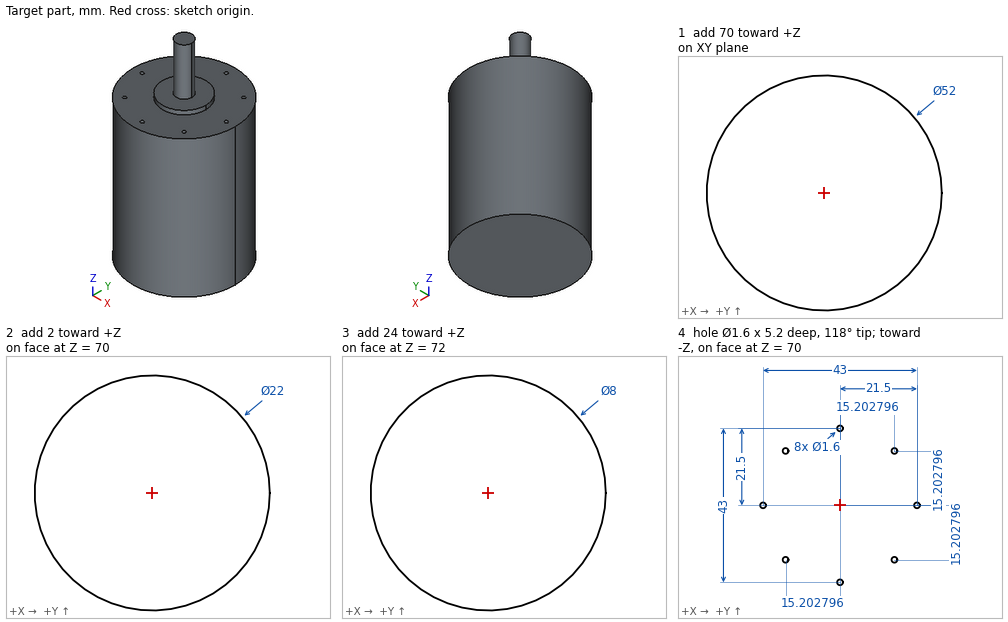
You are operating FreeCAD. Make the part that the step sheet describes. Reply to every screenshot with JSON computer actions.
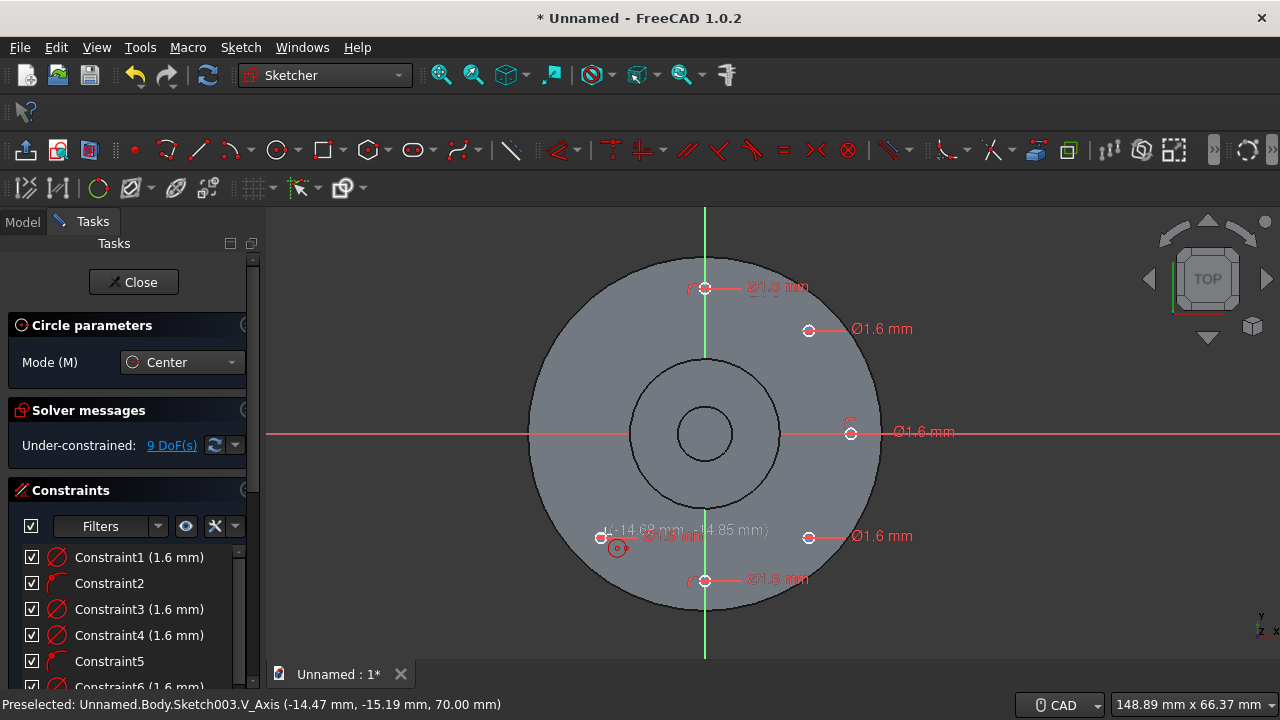
{"action": "scroll", "coordinate": [559, 434], "scroll_direction": "up", "scroll_amount": 8}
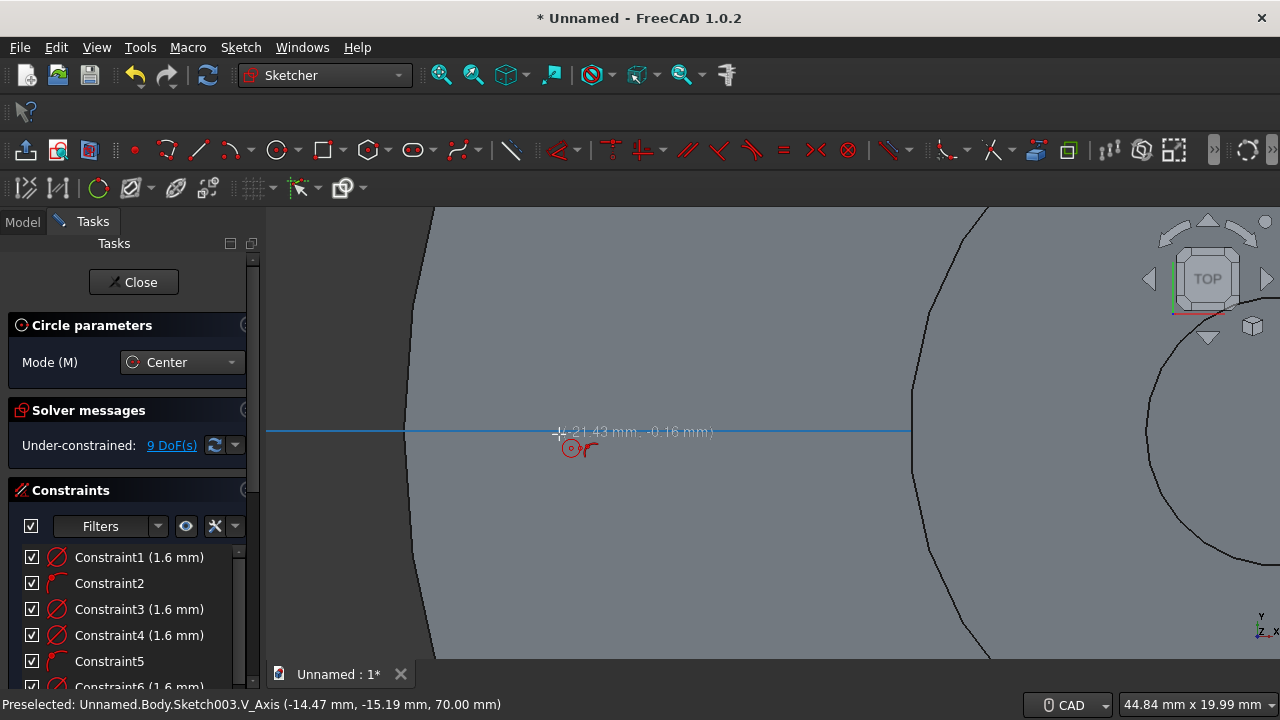
{"action": "scroll", "coordinate": [559, 433], "scroll_direction": "down", "scroll_amount": 8}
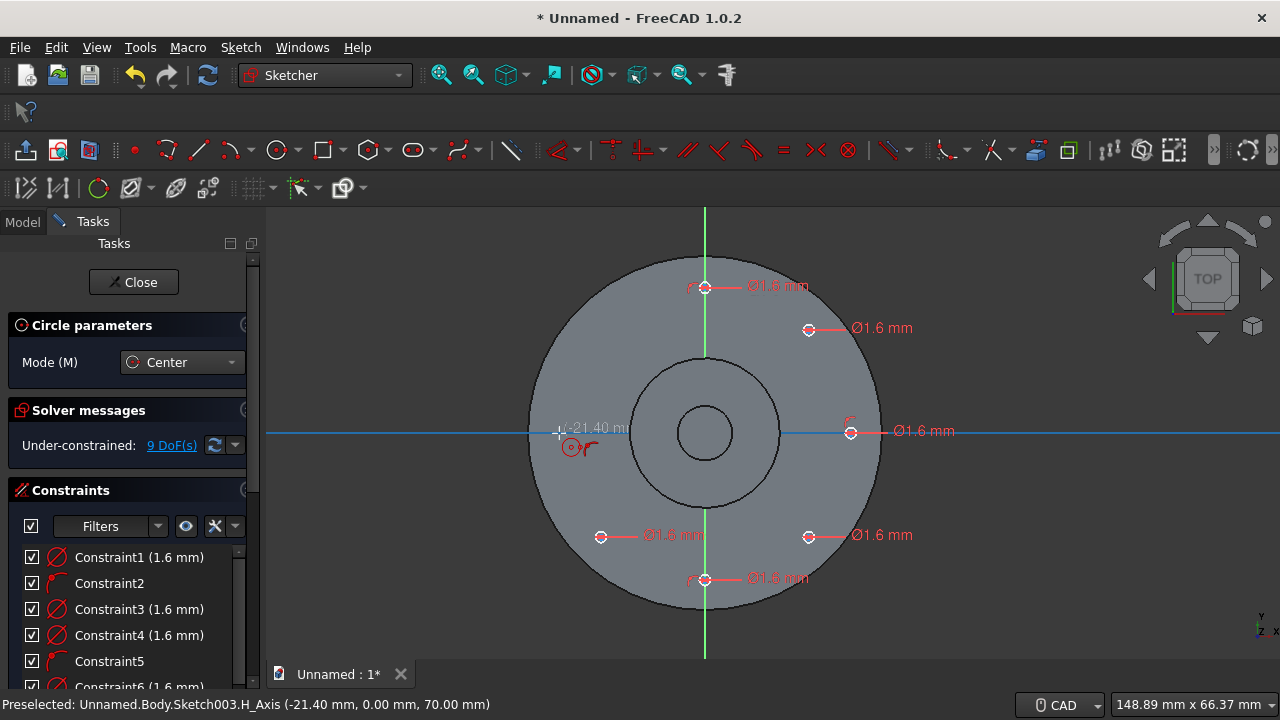
{"action": "left_click", "coordinate": [559, 433]}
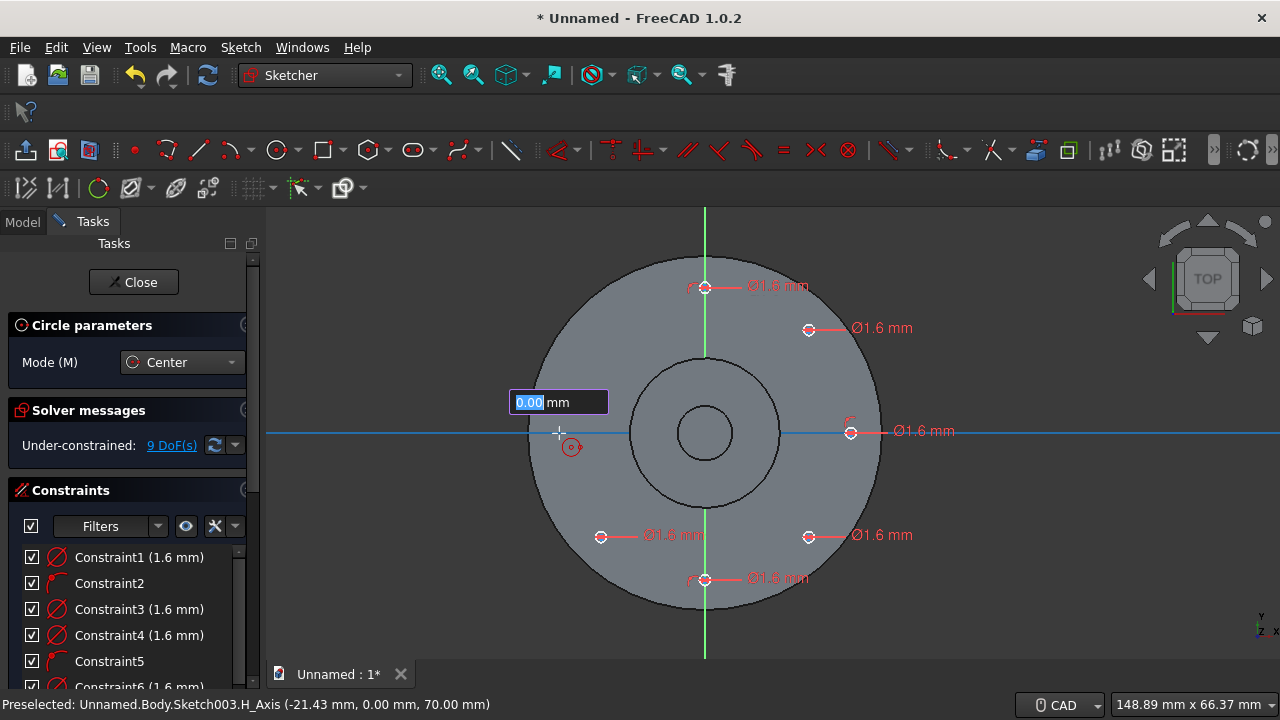
{"action": "scroll", "coordinate": [557, 438], "scroll_direction": "up", "scroll_amount": 6}
{"action": "mouse_move", "coordinate": [555, 438]}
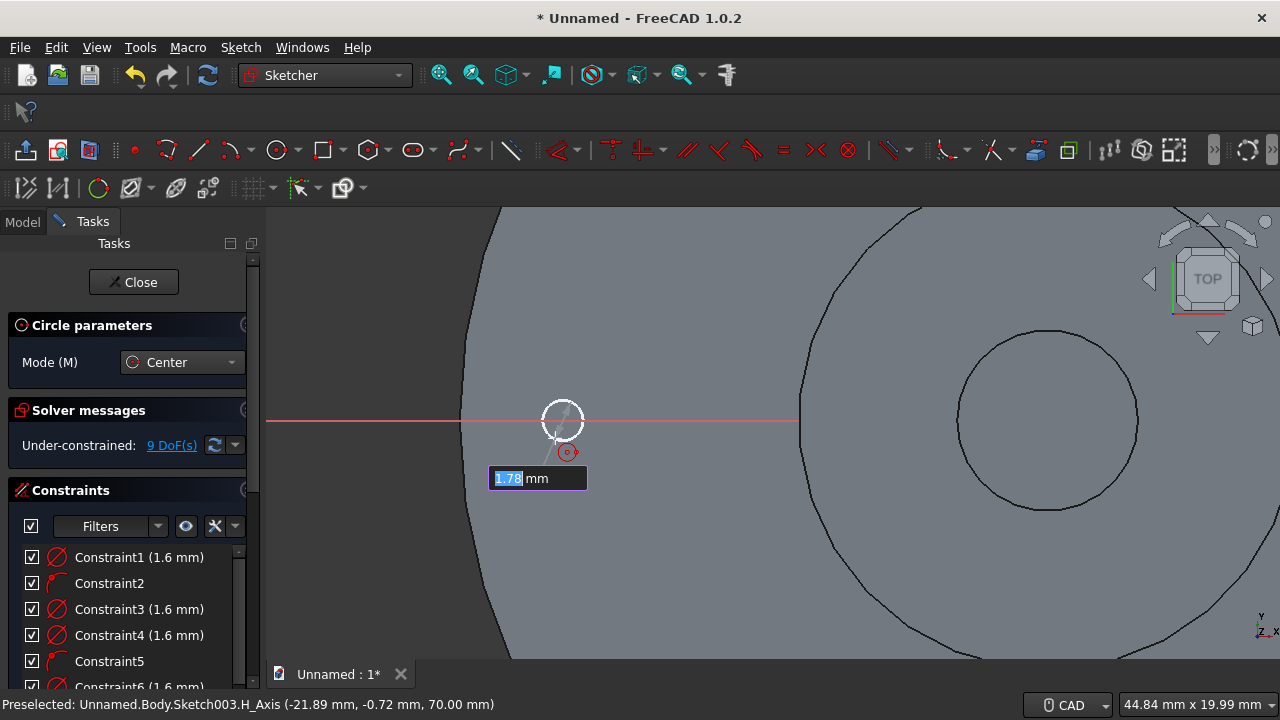
{"action": "type", "text": "1.6"}
{"action": "key", "text": "Return"}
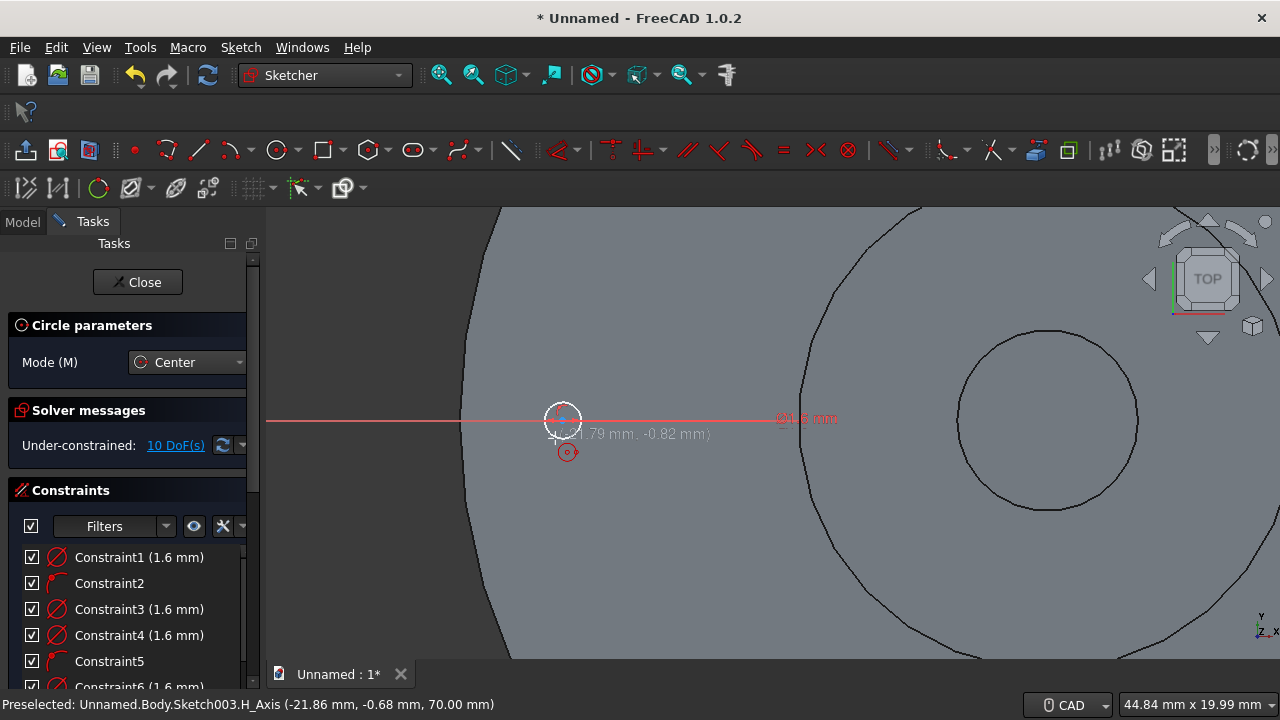
{"action": "scroll", "coordinate": [557, 438], "scroll_direction": "down", "scroll_amount": 6}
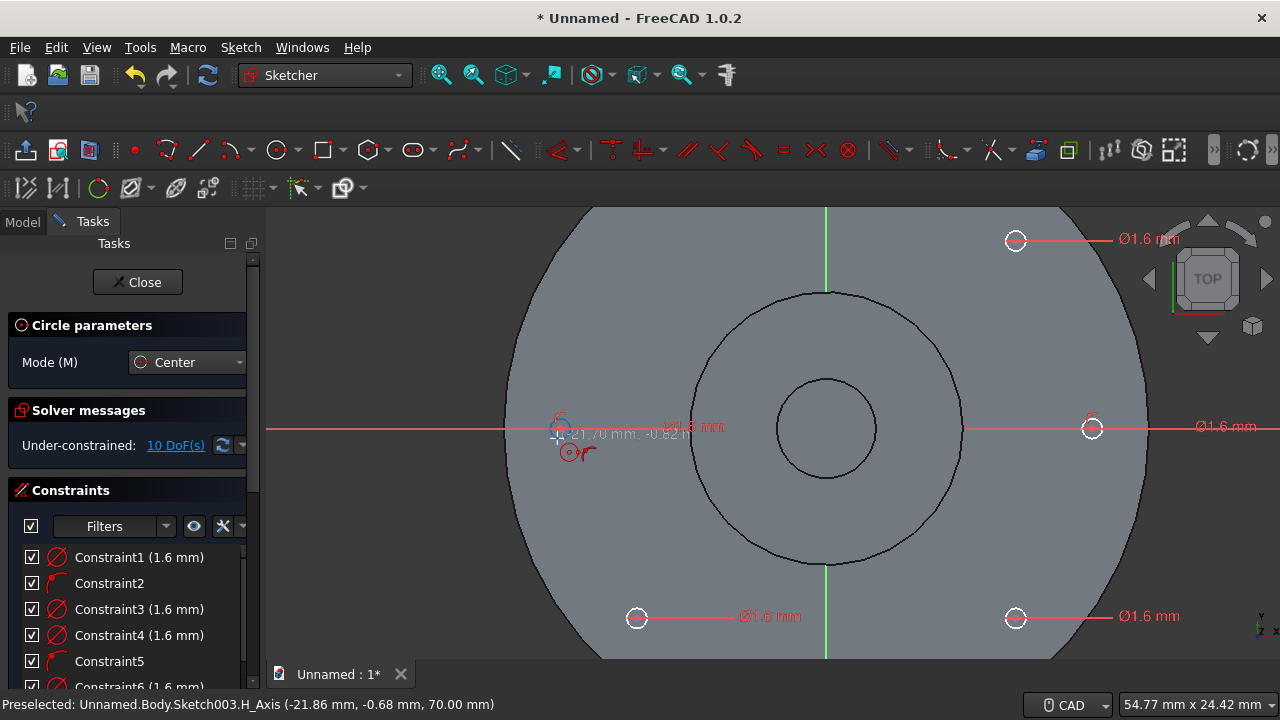
{"action": "scroll", "coordinate": [601, 330], "scroll_direction": "up", "scroll_amount": 8}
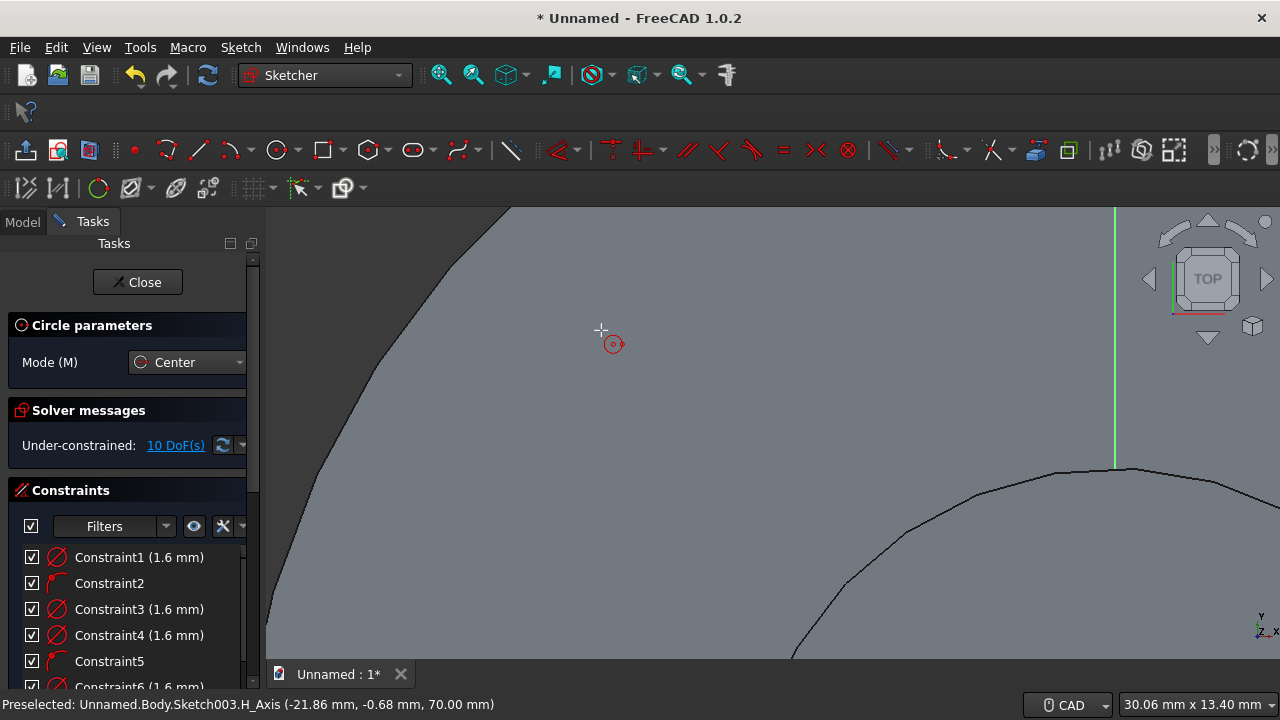
{"action": "scroll", "coordinate": [601, 330], "scroll_direction": "down", "scroll_amount": 8}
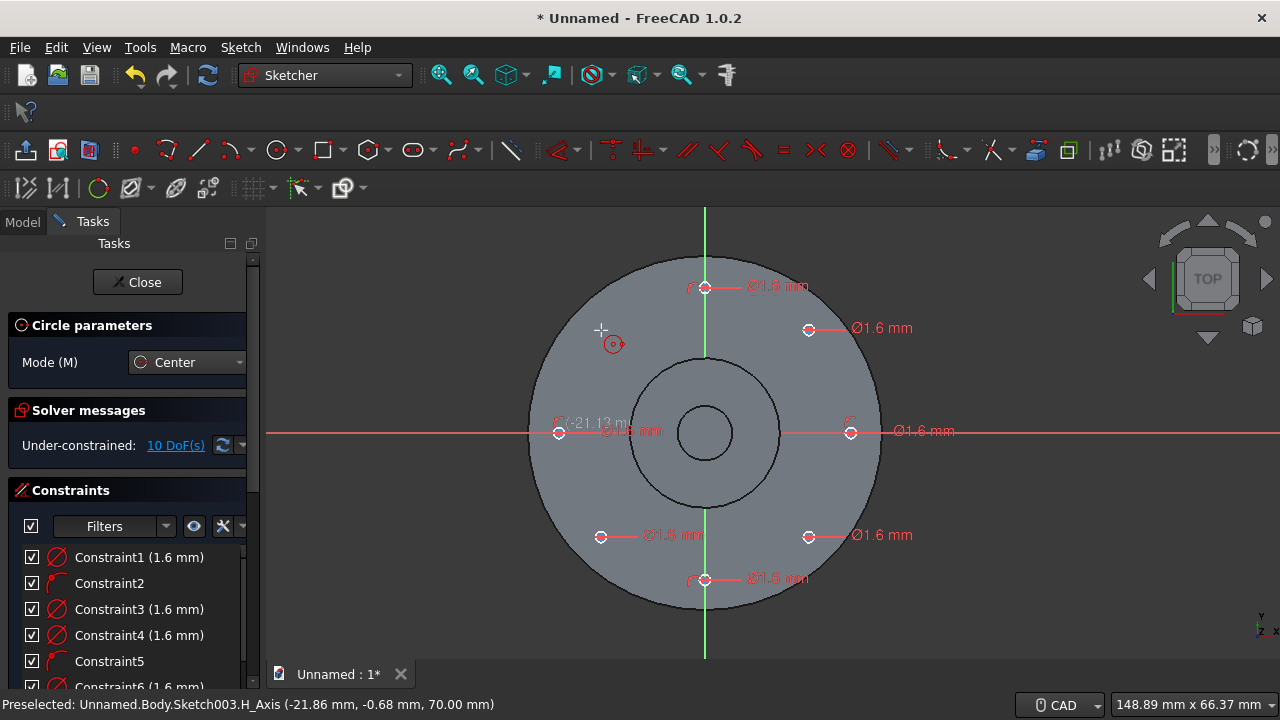
{"action": "left_click", "coordinate": [601, 330]}
{"action": "mouse_move", "coordinate": [605, 326]}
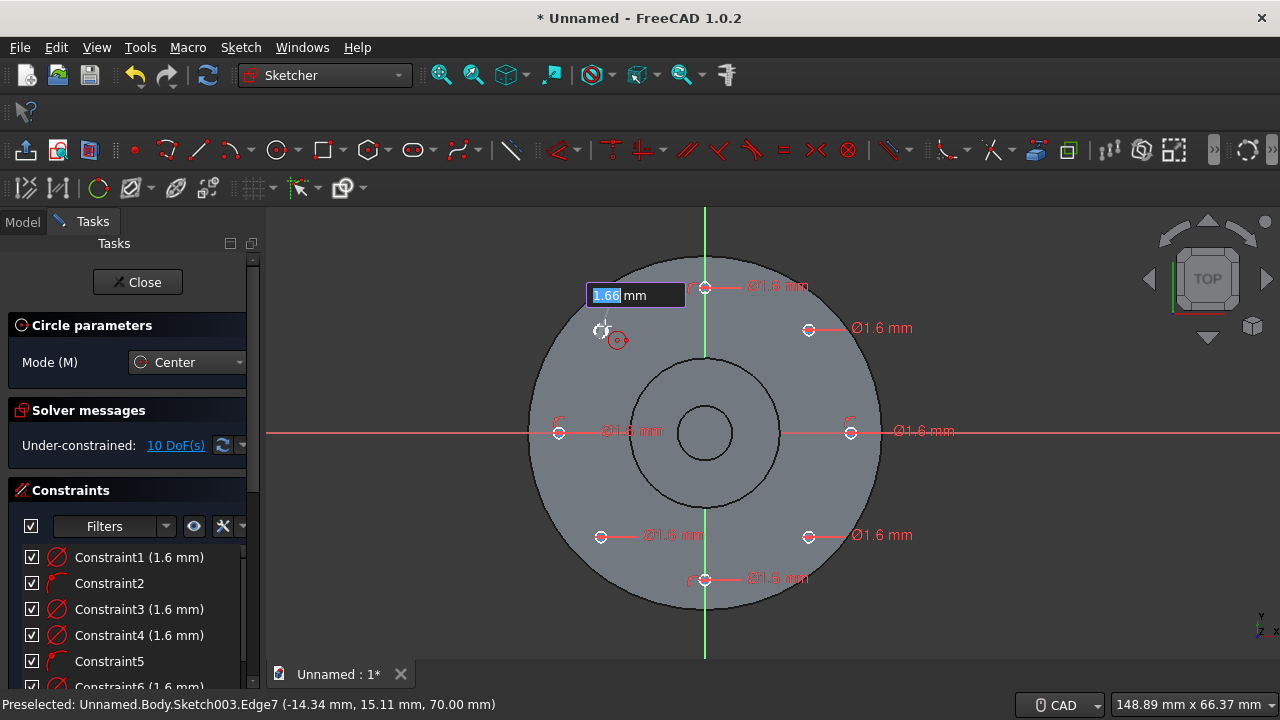
{"action": "type", "text": "1.6"}
{"action": "key", "text": "Return"}
{"action": "key", "text": "Escape"}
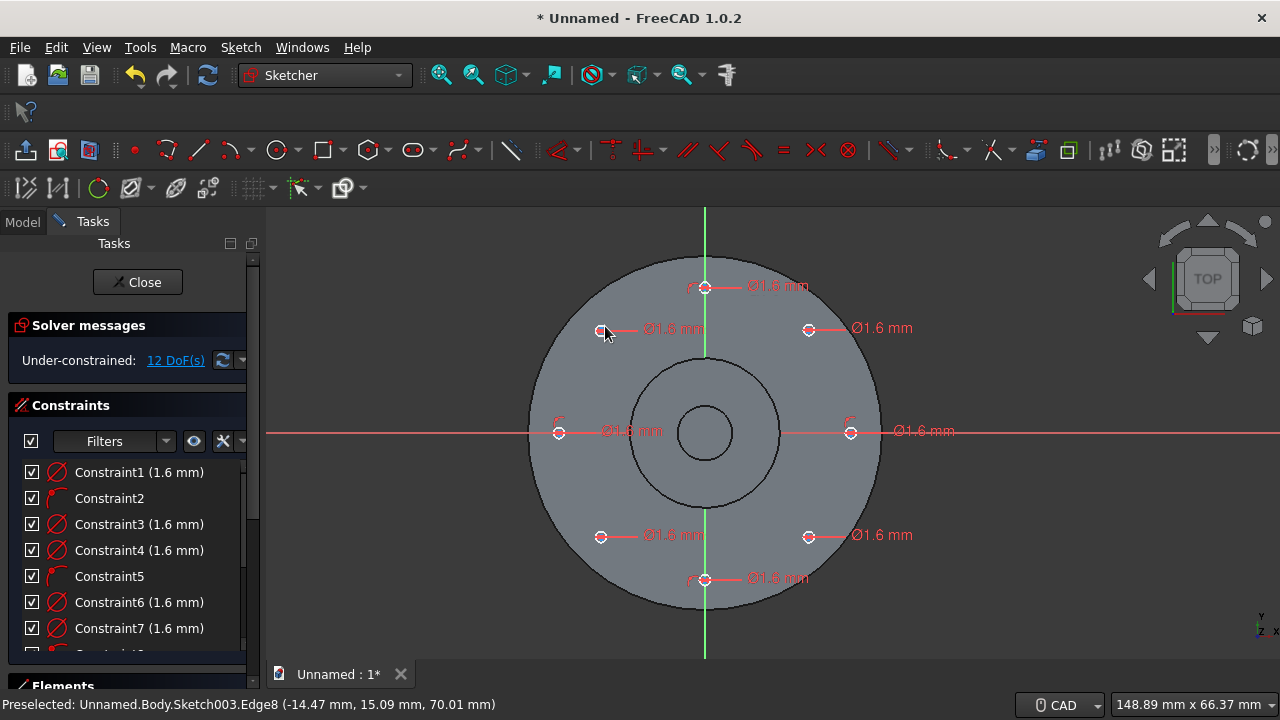
{"action": "left_click", "coordinate": [809, 330]}